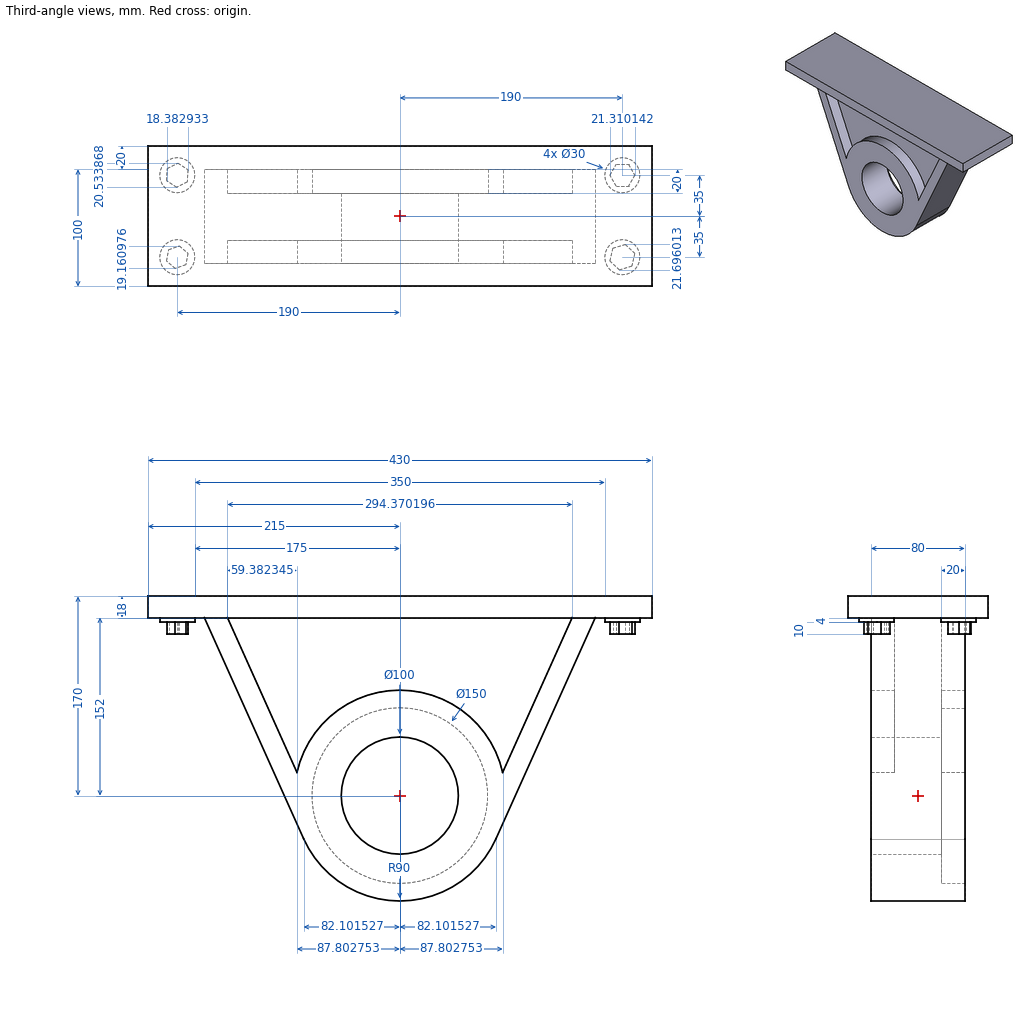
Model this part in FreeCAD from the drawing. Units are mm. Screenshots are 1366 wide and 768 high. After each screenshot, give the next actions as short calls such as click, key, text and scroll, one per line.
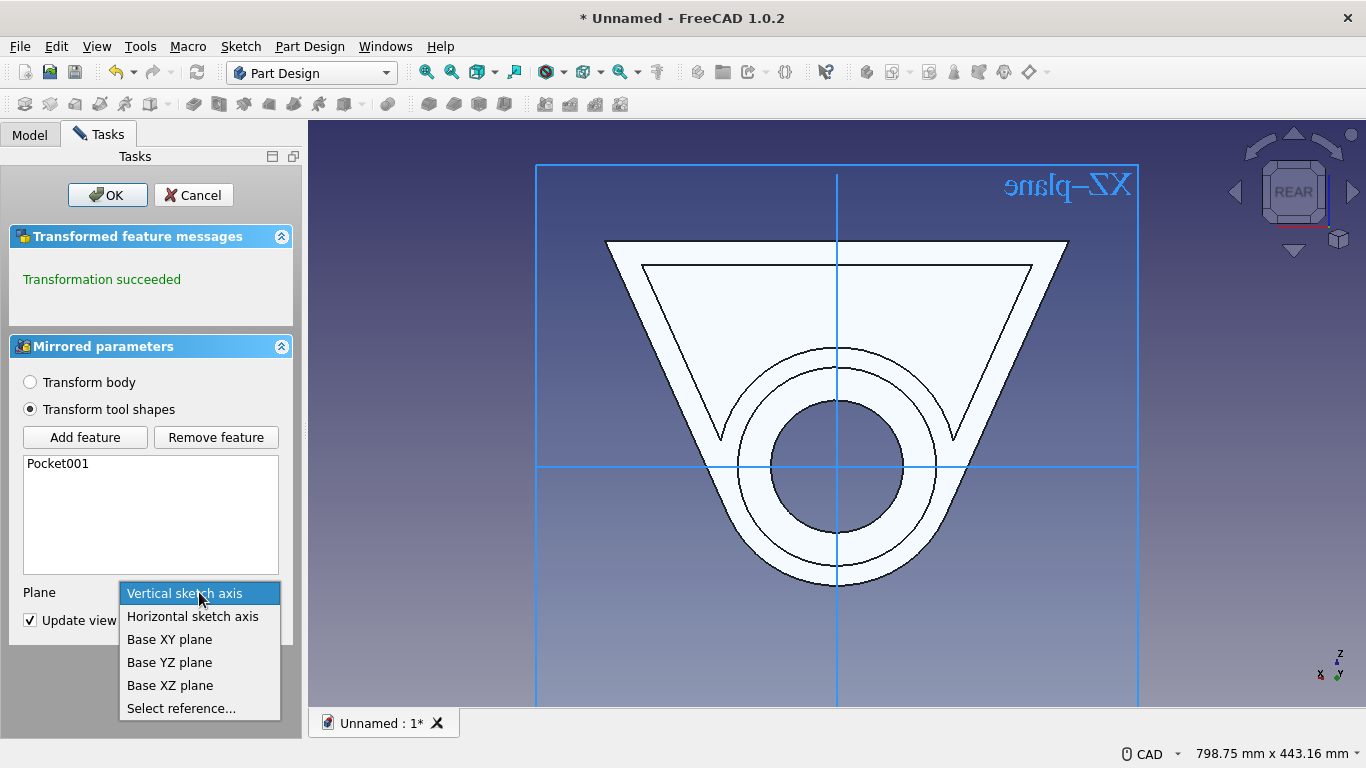
click(198, 686)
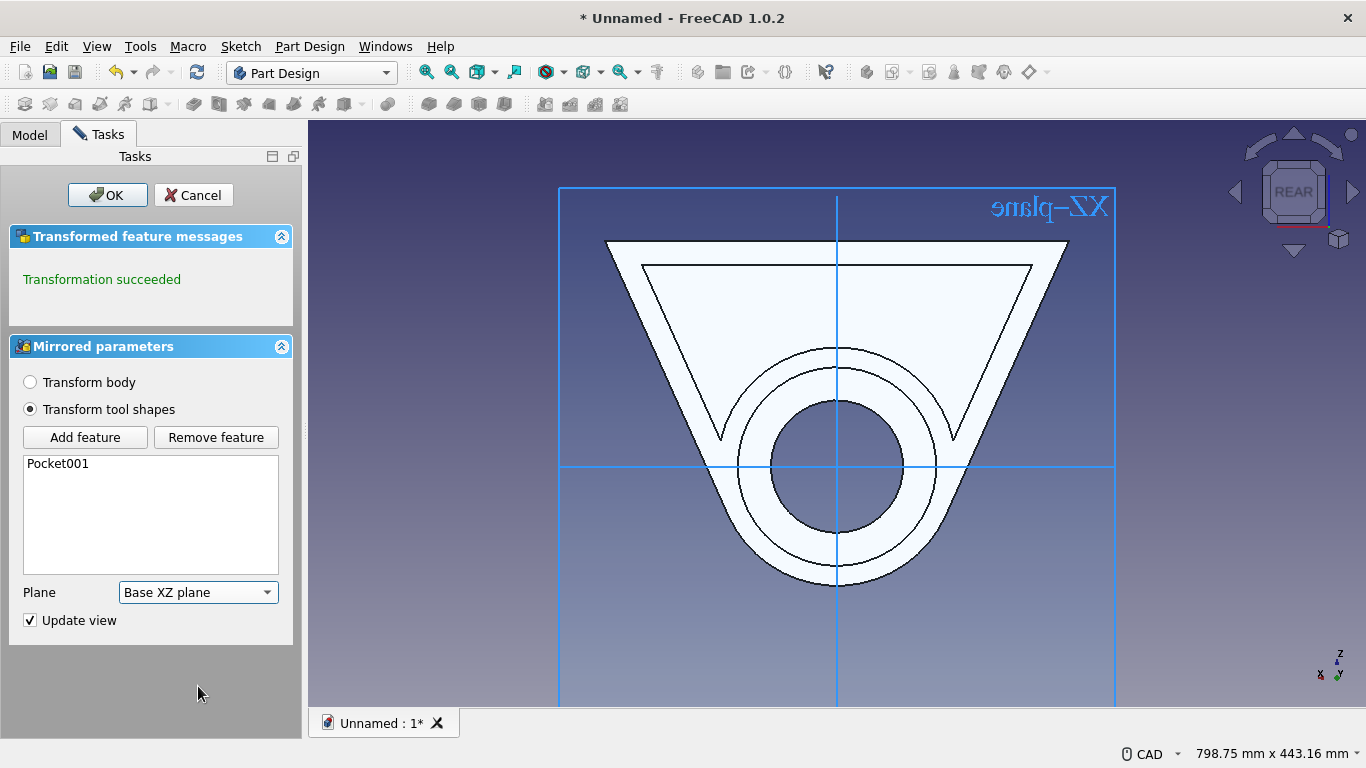
click(108, 195)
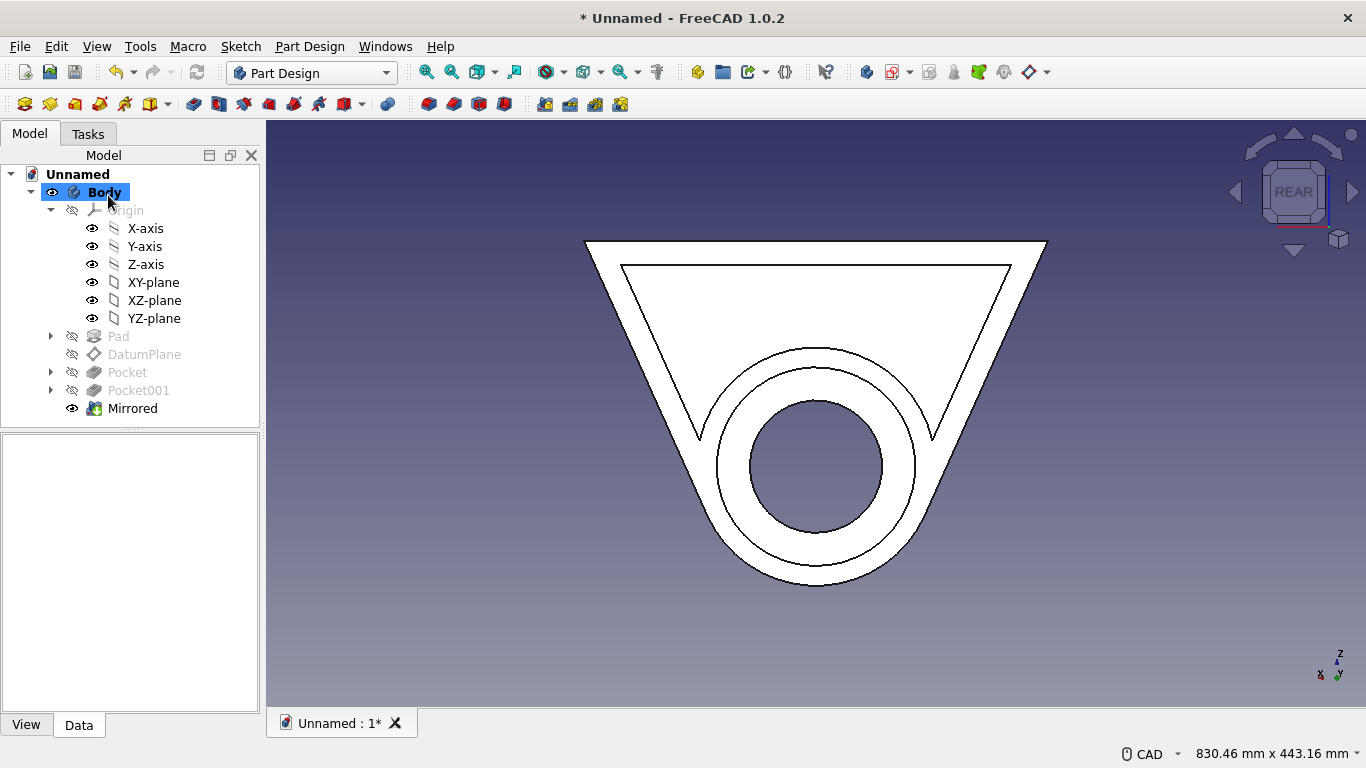
scroll(1015, 265, up, 6)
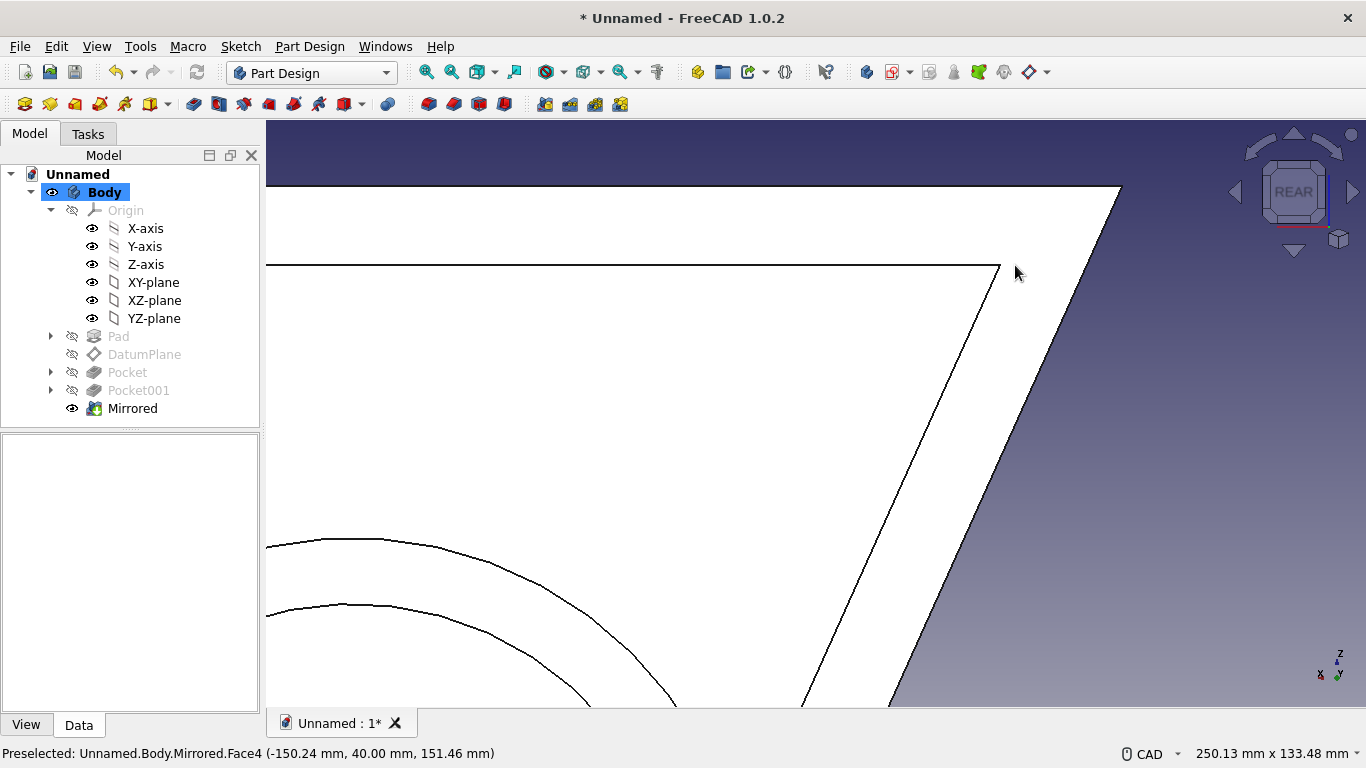
click(1012, 267)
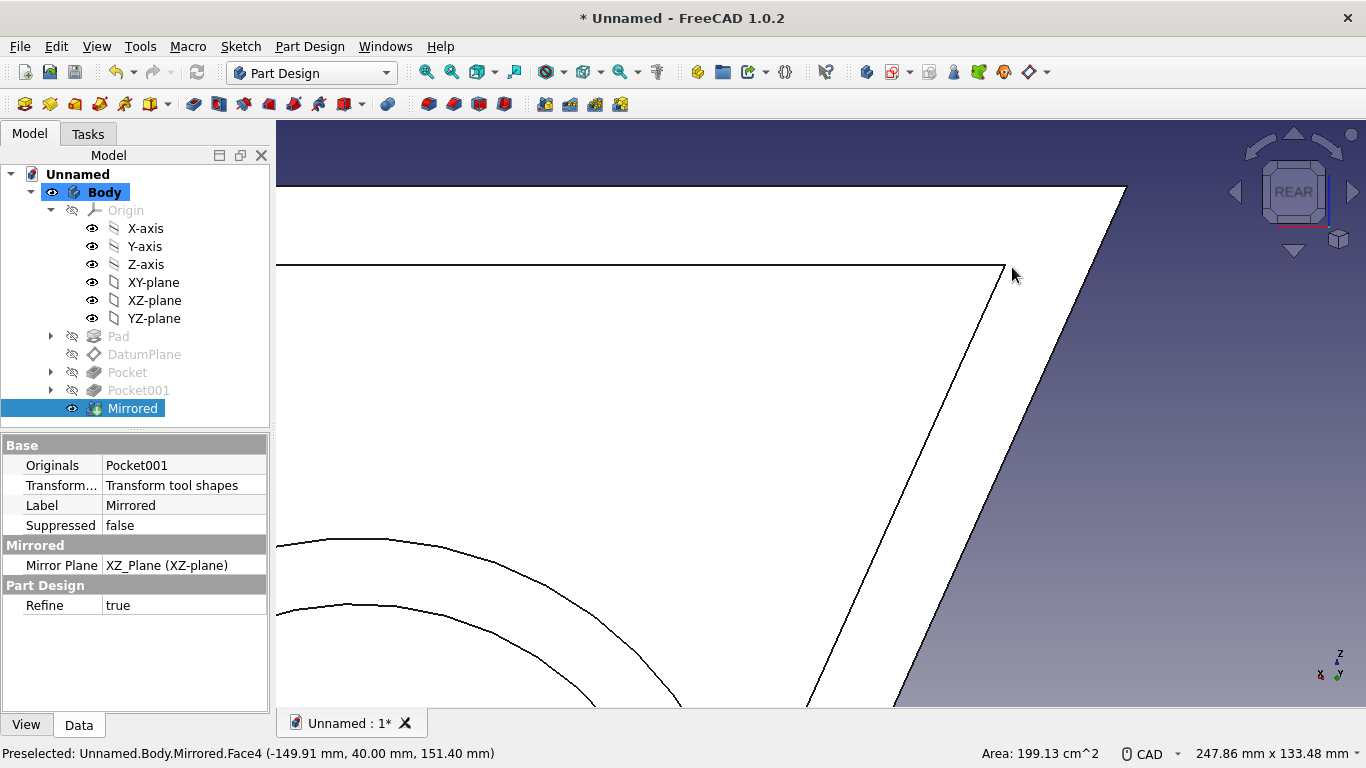
click(892, 72)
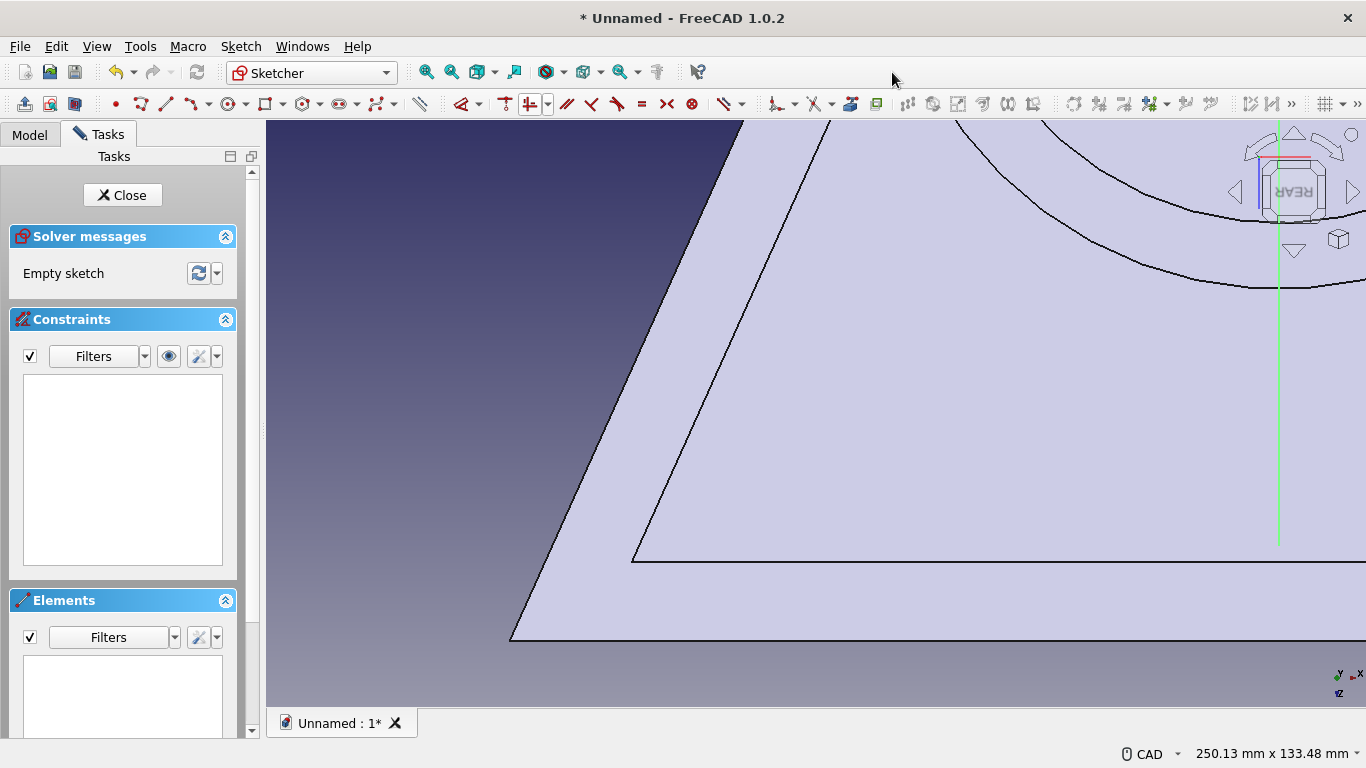
scroll(438, 499, down, 5)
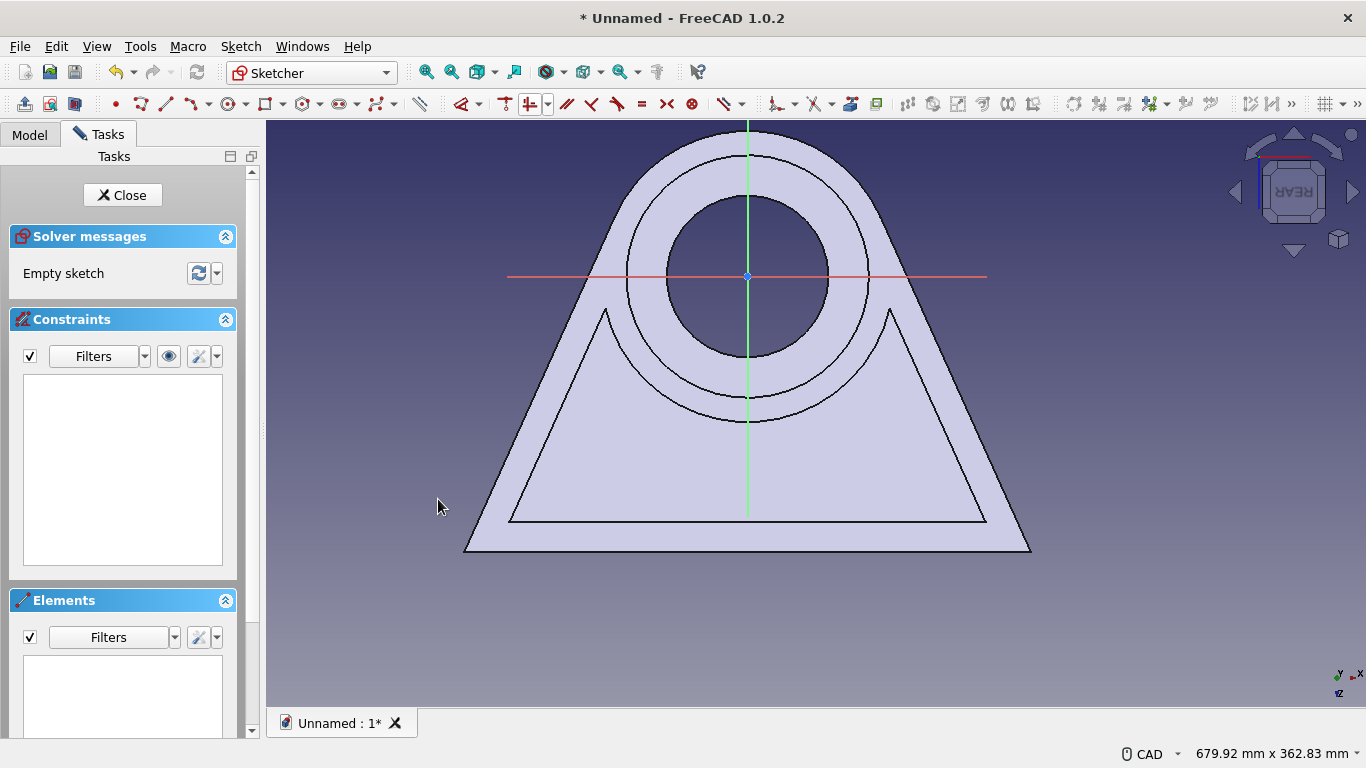
click(264, 104)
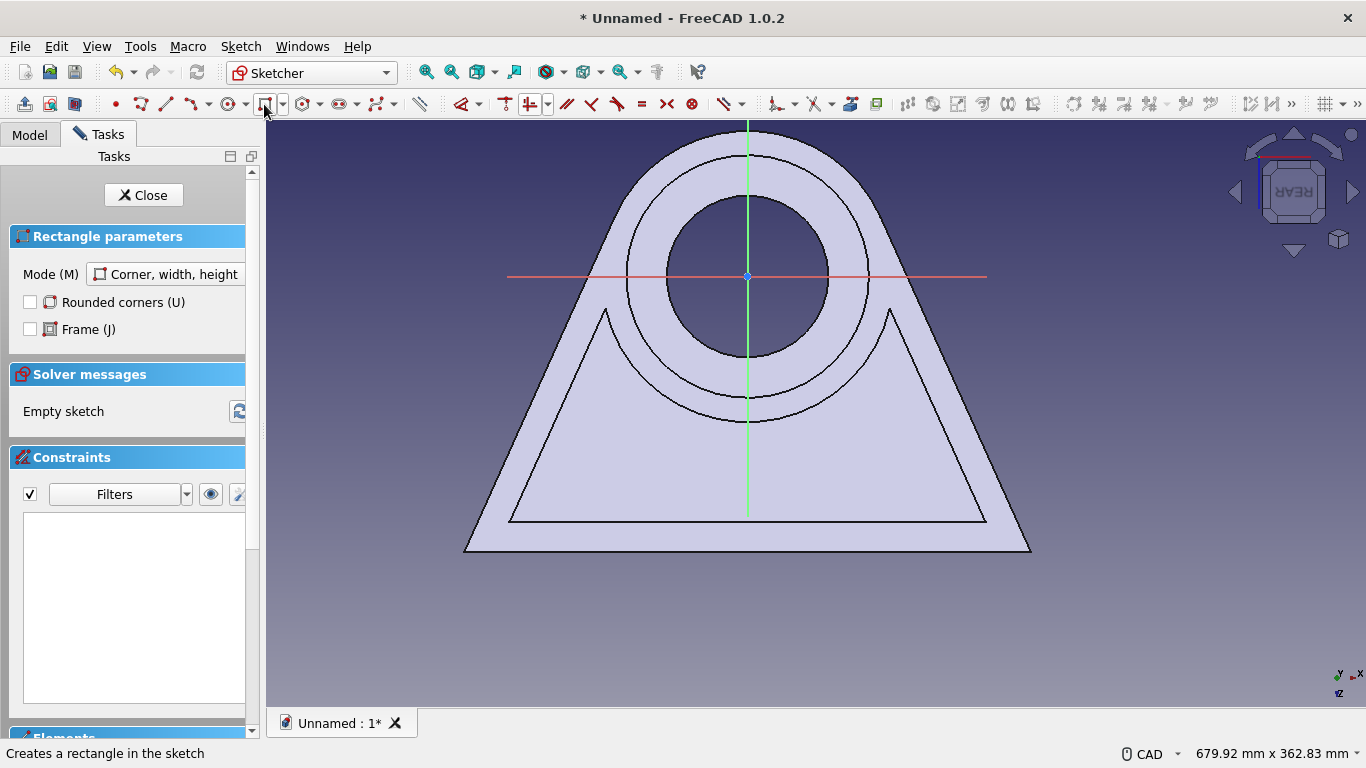
click(400, 522)
click(1095, 552)
key(Escape)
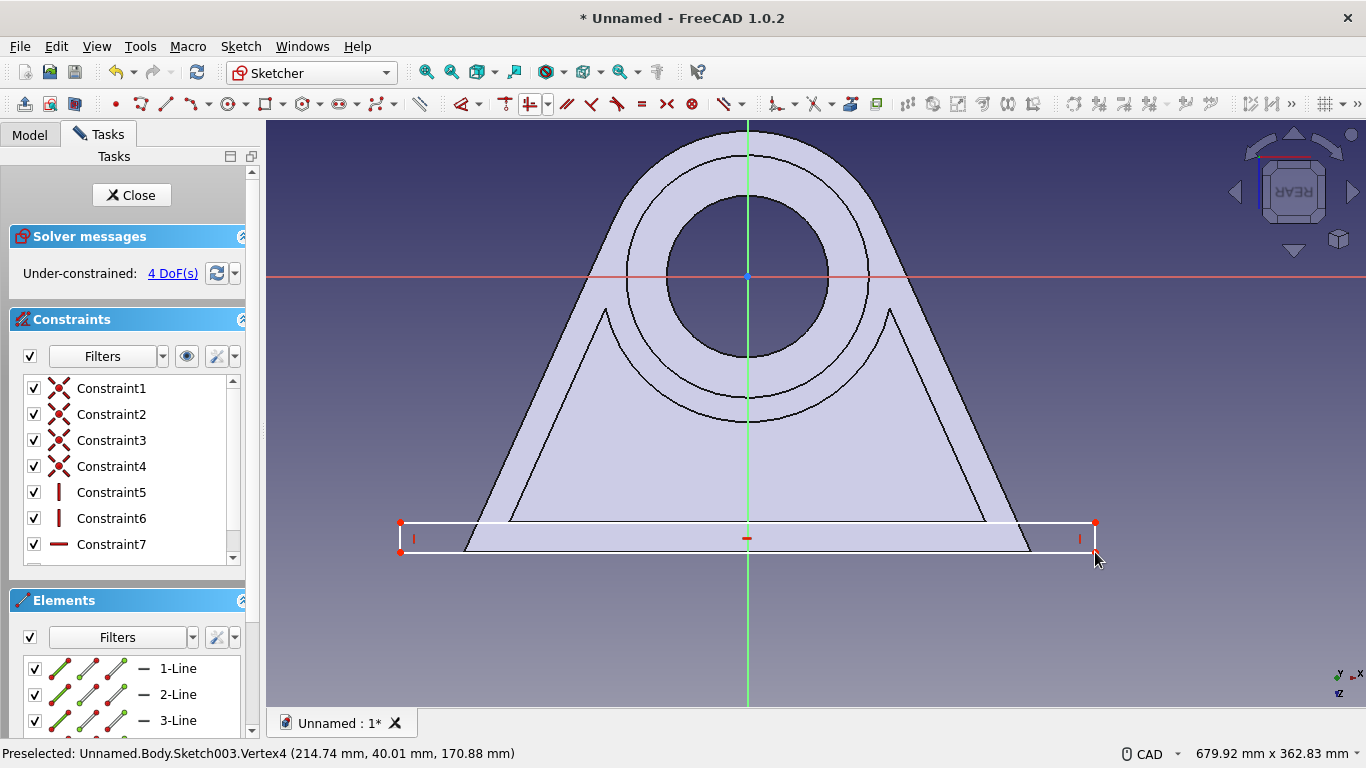
click(460, 104)